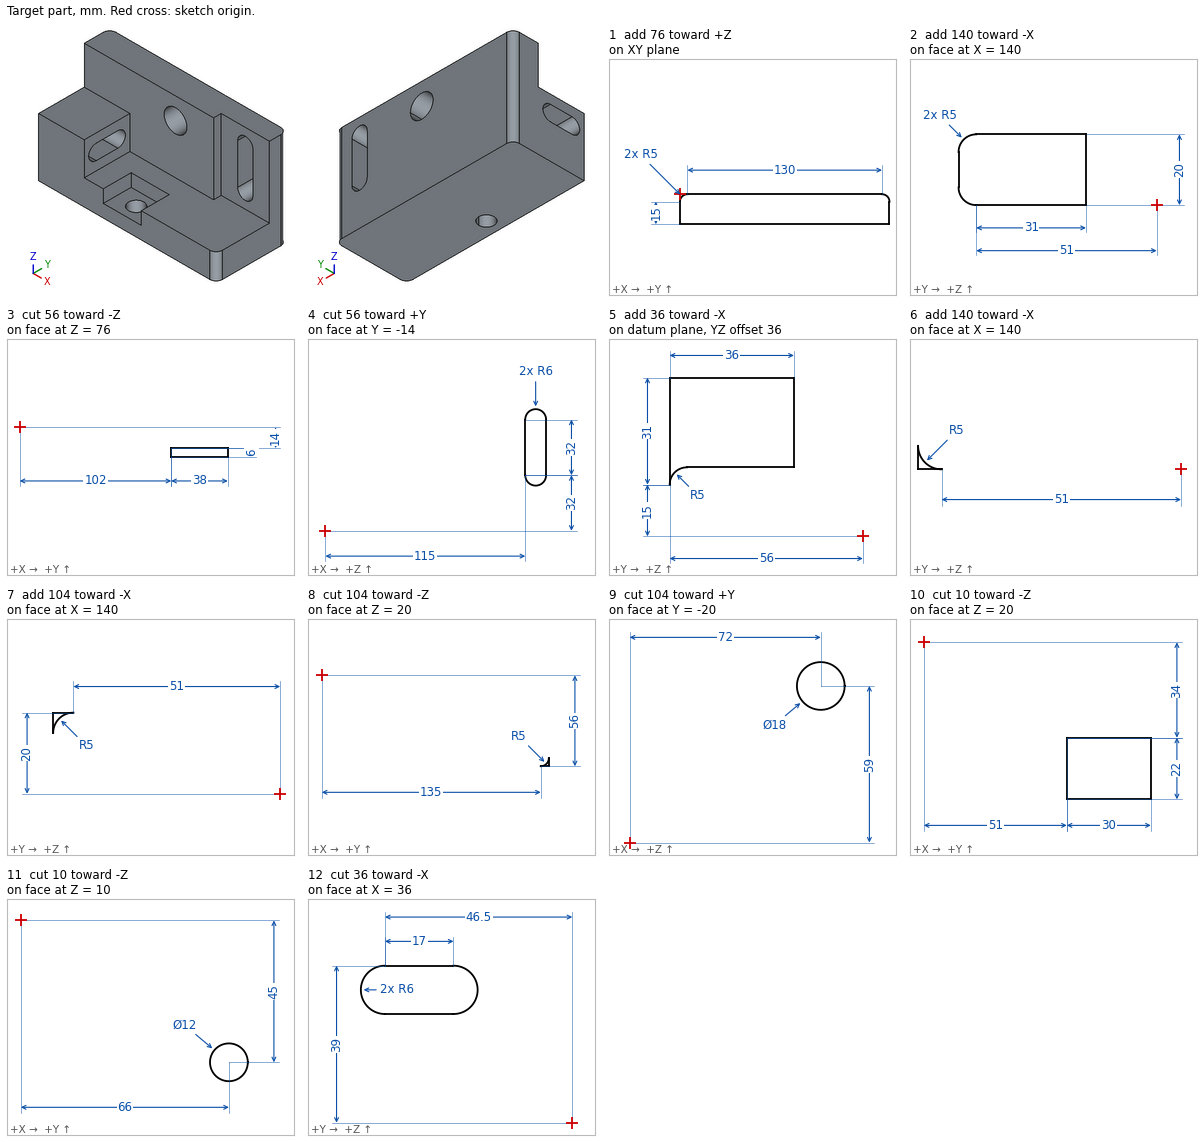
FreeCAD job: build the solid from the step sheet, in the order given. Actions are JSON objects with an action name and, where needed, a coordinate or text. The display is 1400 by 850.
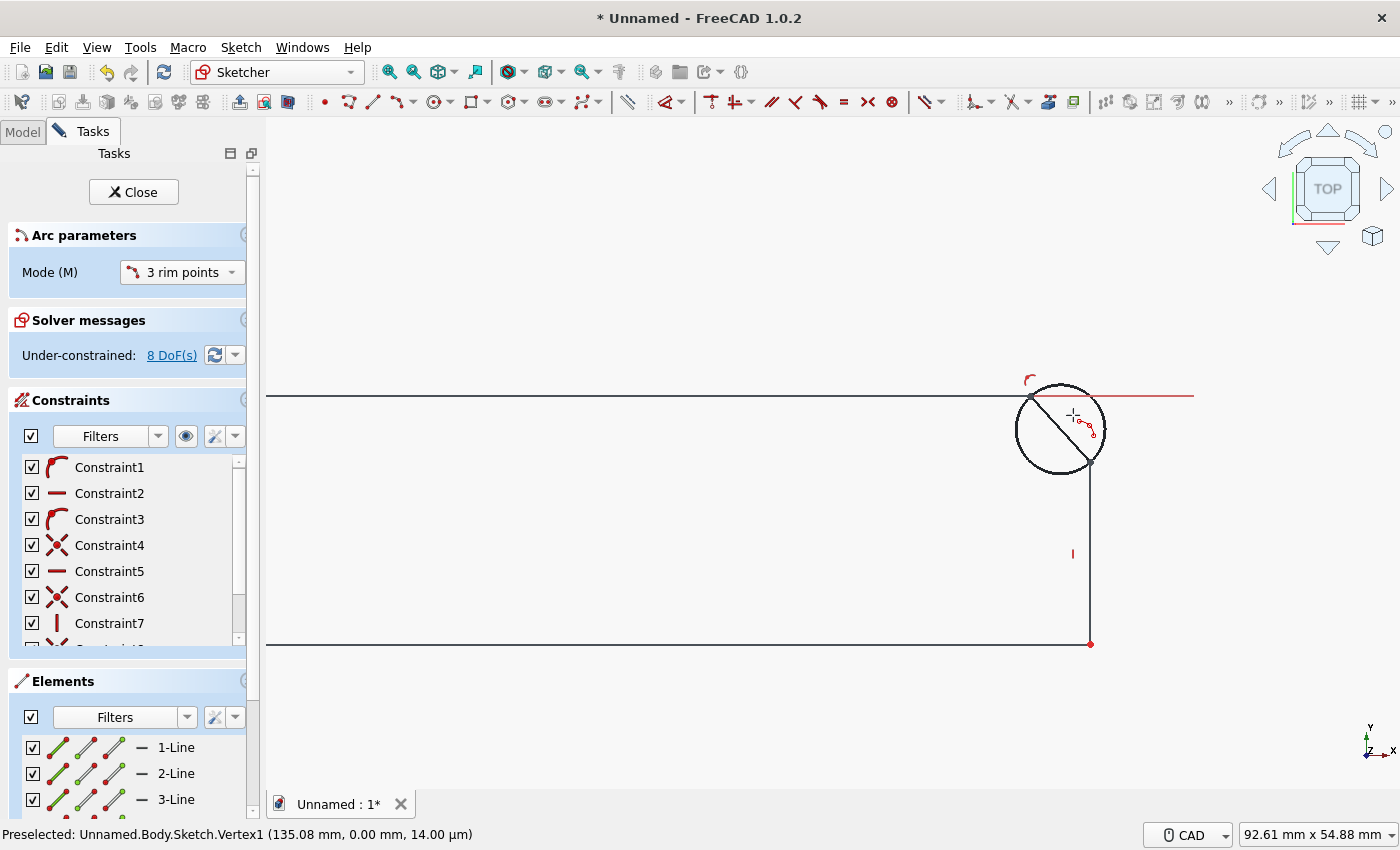
{"action": "left_click", "coordinate": [1073, 414]}
{"action": "key", "text": "Escape"}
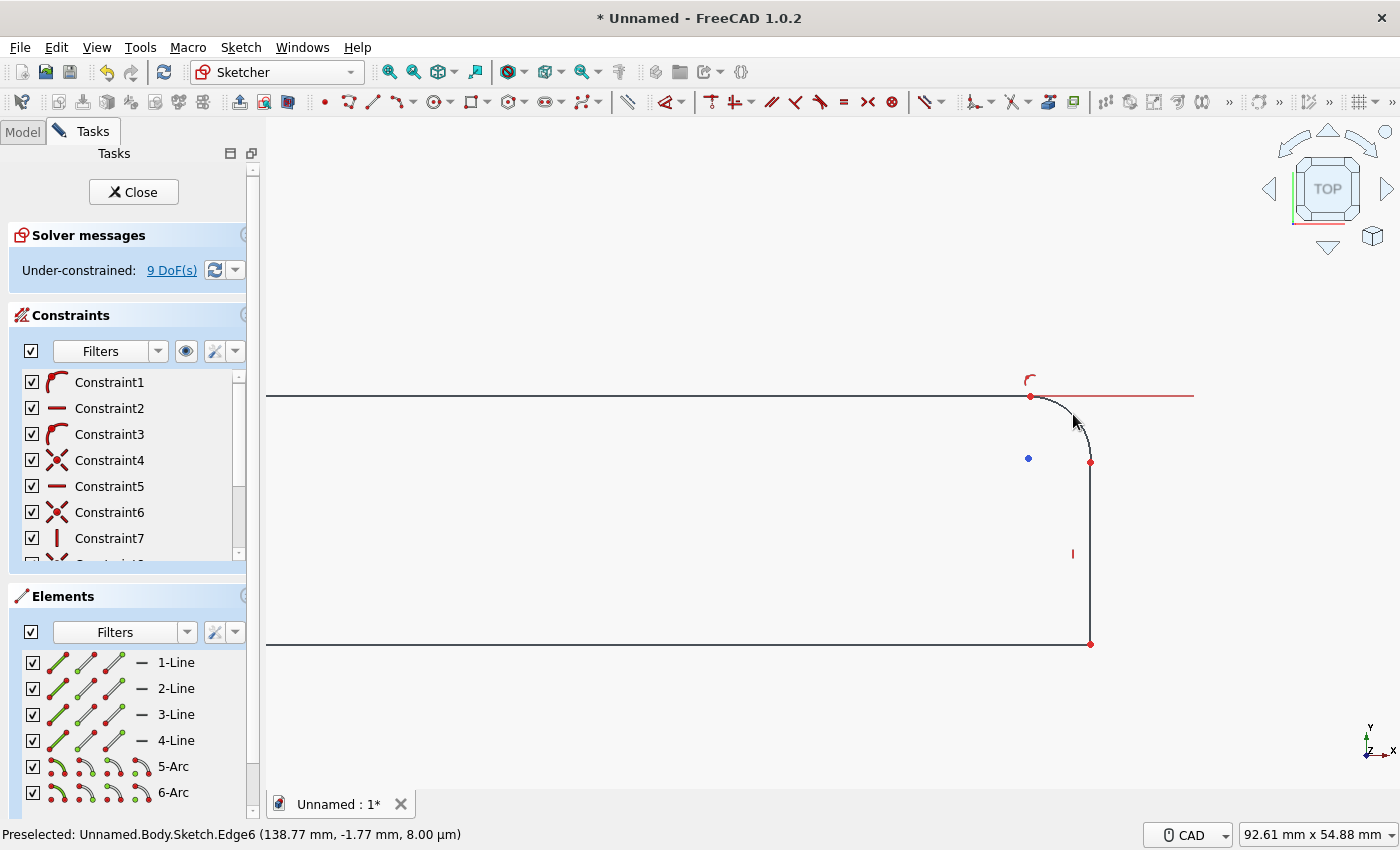
{"action": "left_click", "coordinate": [553, 396]}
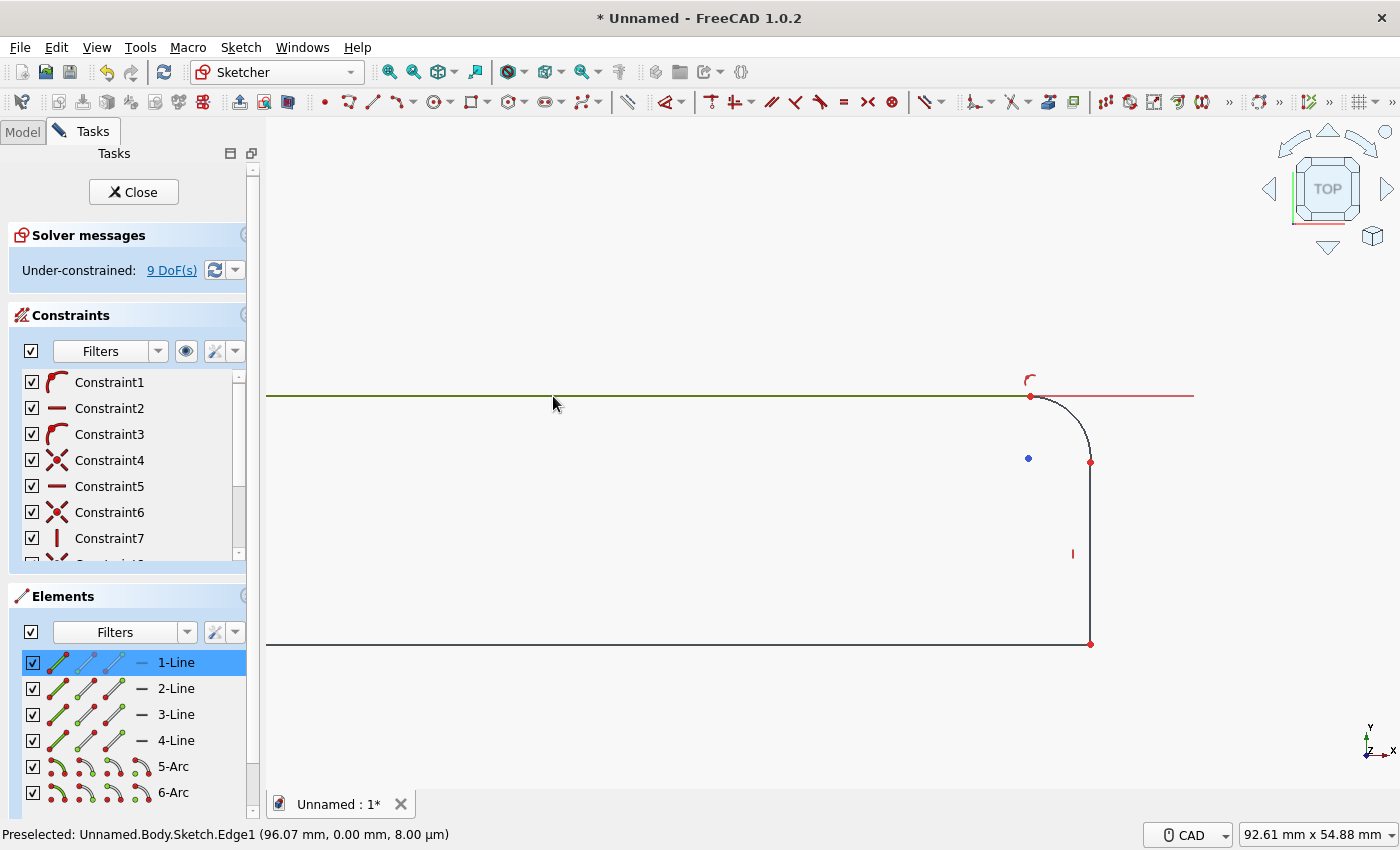
{"action": "scroll", "coordinate": [1073, 415], "scroll_direction": "down", "scroll_amount": 5}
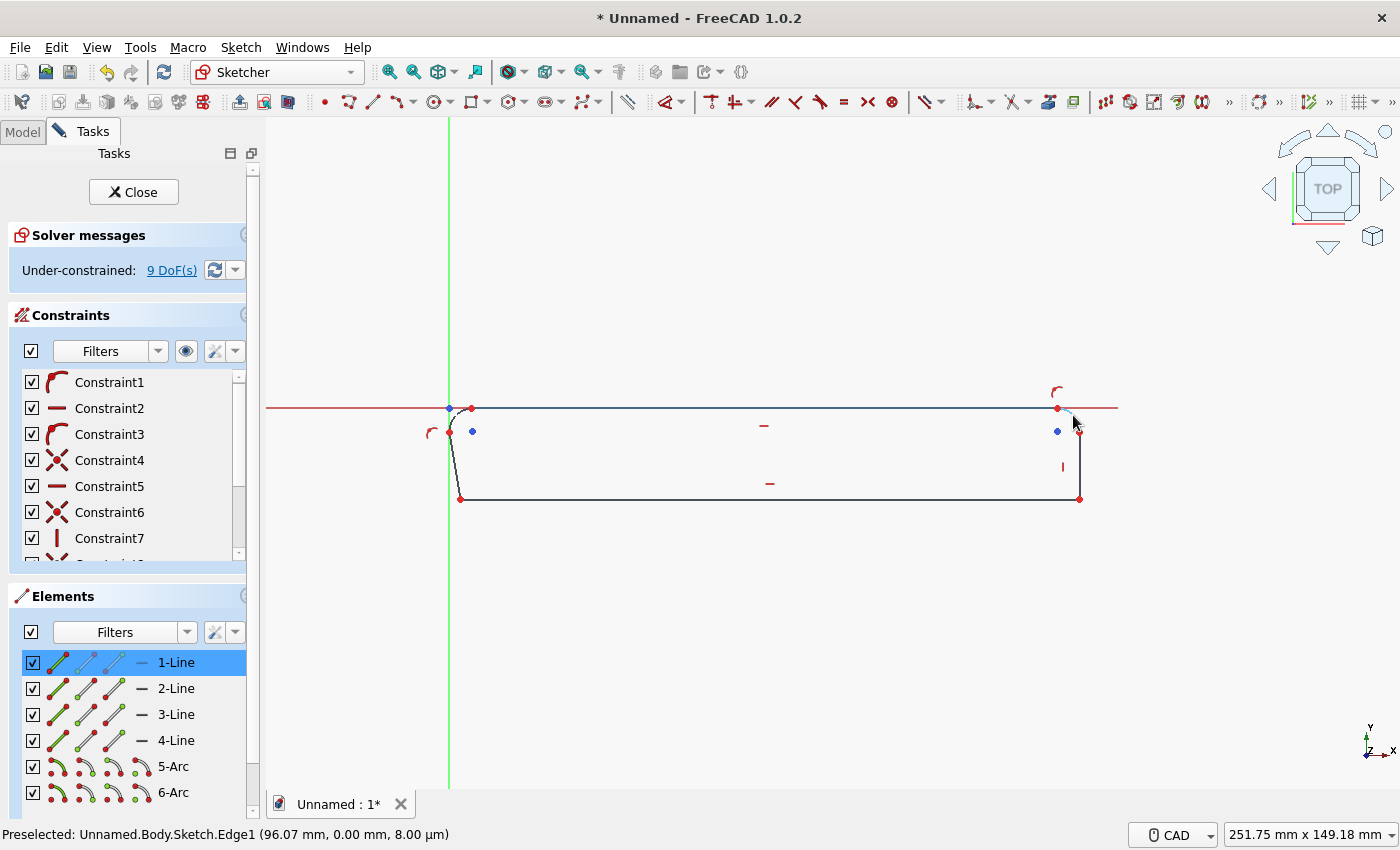
{"action": "scroll", "coordinate": [456, 416], "scroll_direction": "up", "scroll_amount": 5}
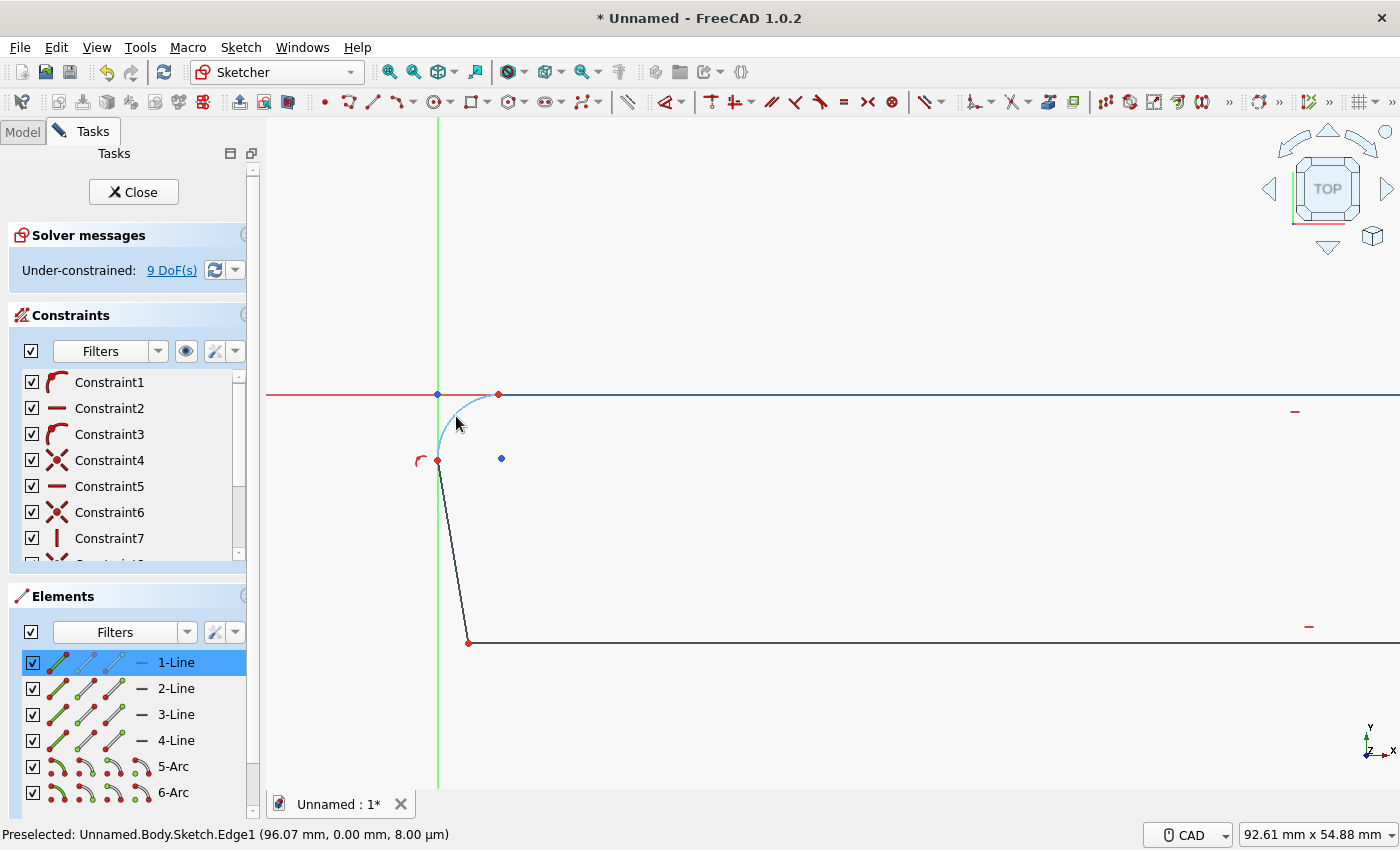
{"action": "left_click", "coordinate": [455, 415]}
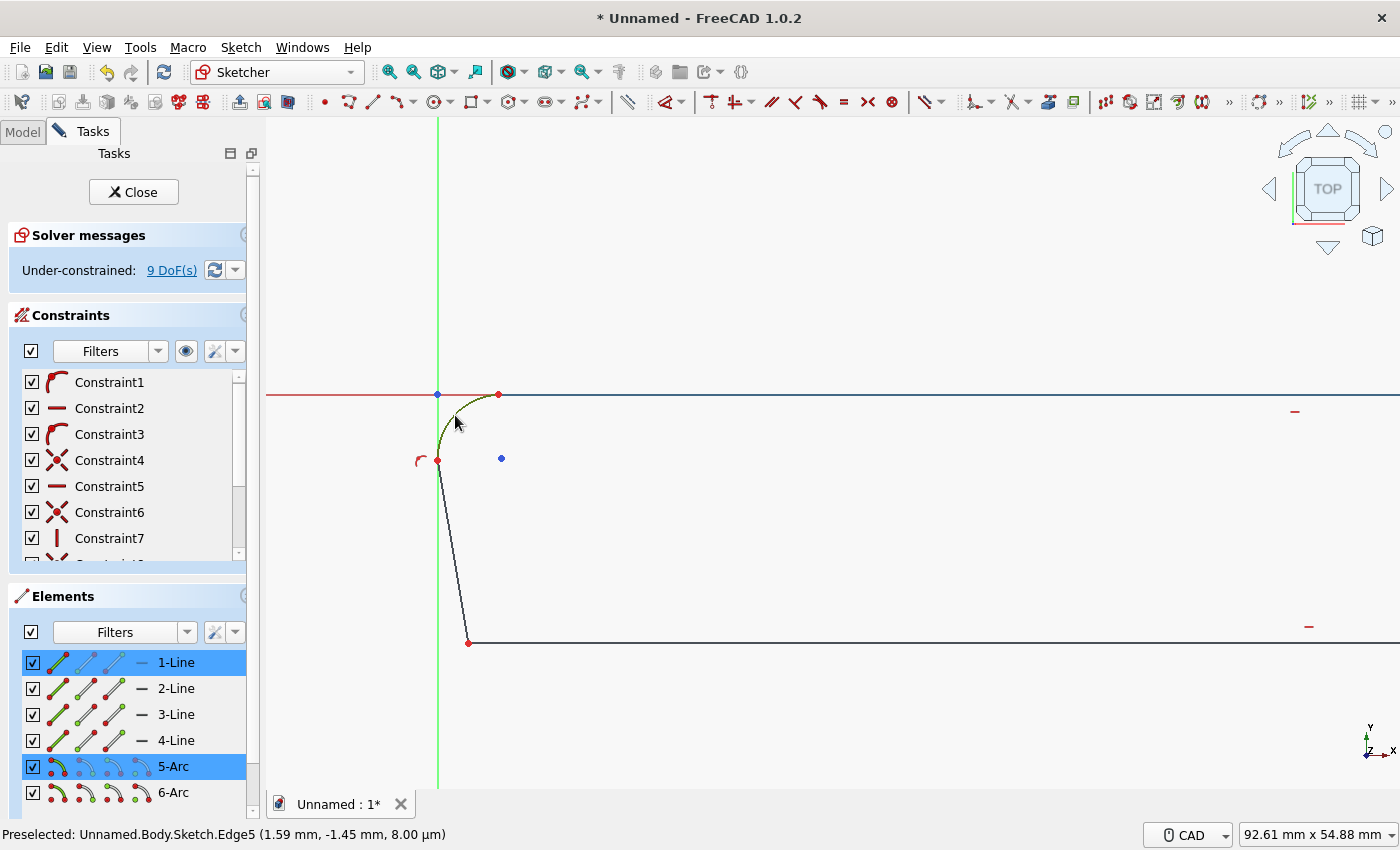
{"action": "left_click", "coordinate": [820, 102]}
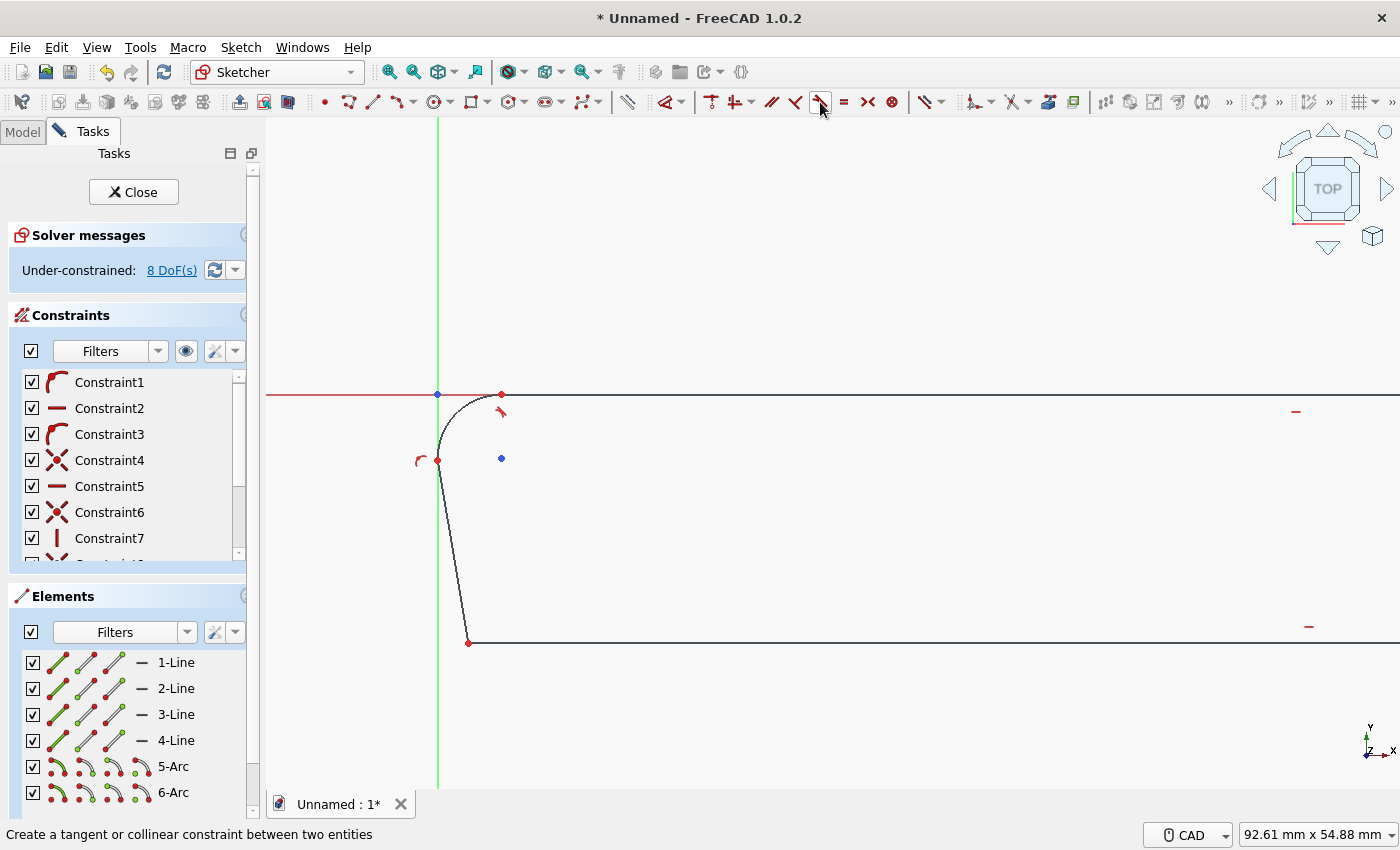
{"action": "left_click", "coordinate": [979, 395]}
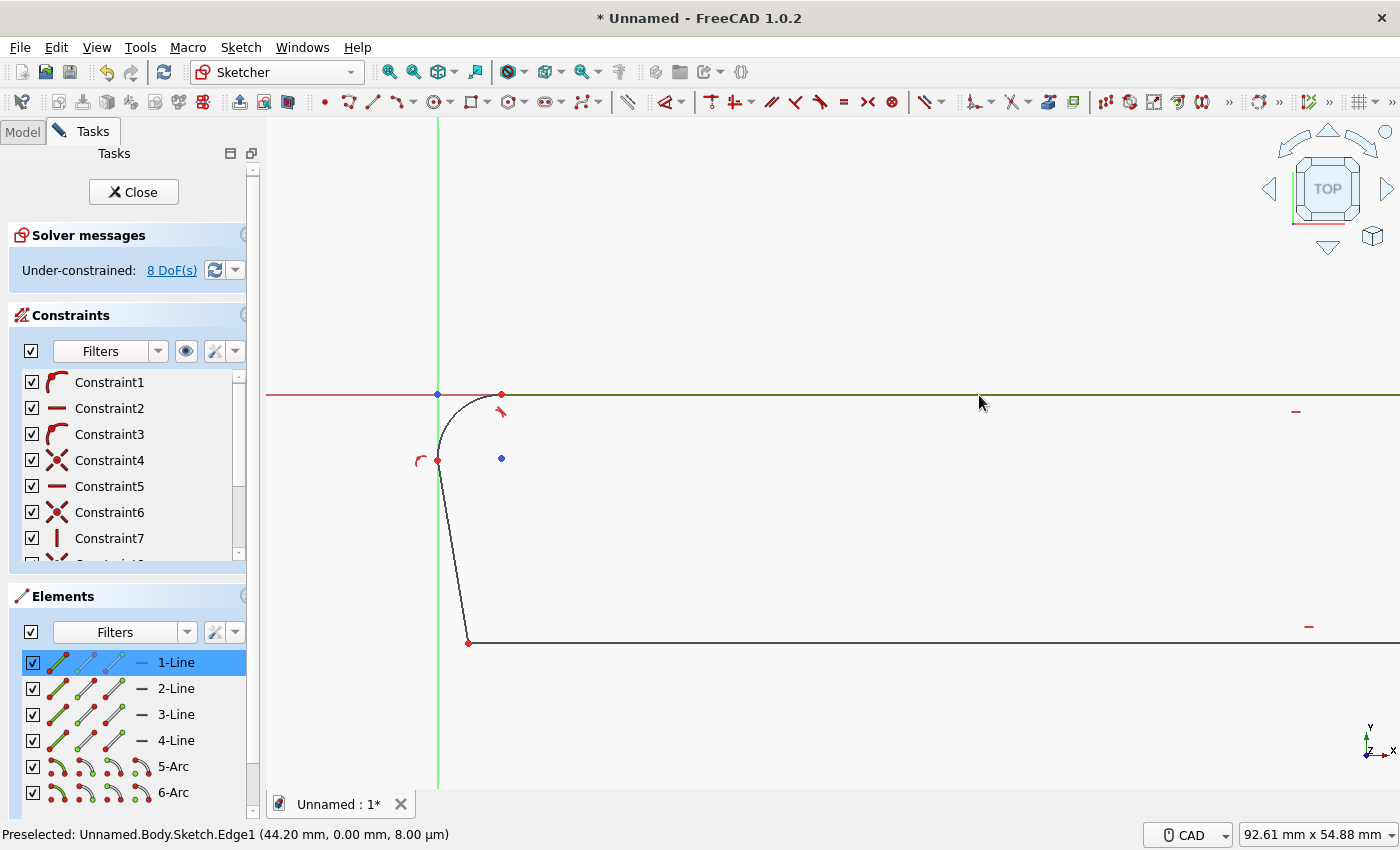
{"action": "scroll", "coordinate": [456, 416], "scroll_direction": "down", "scroll_amount": 5}